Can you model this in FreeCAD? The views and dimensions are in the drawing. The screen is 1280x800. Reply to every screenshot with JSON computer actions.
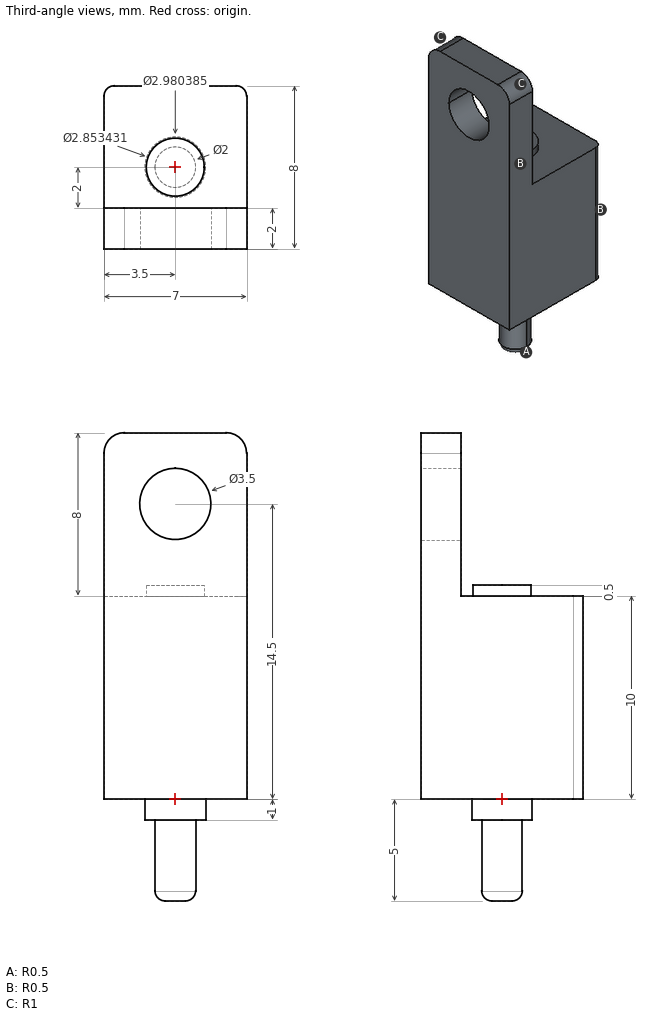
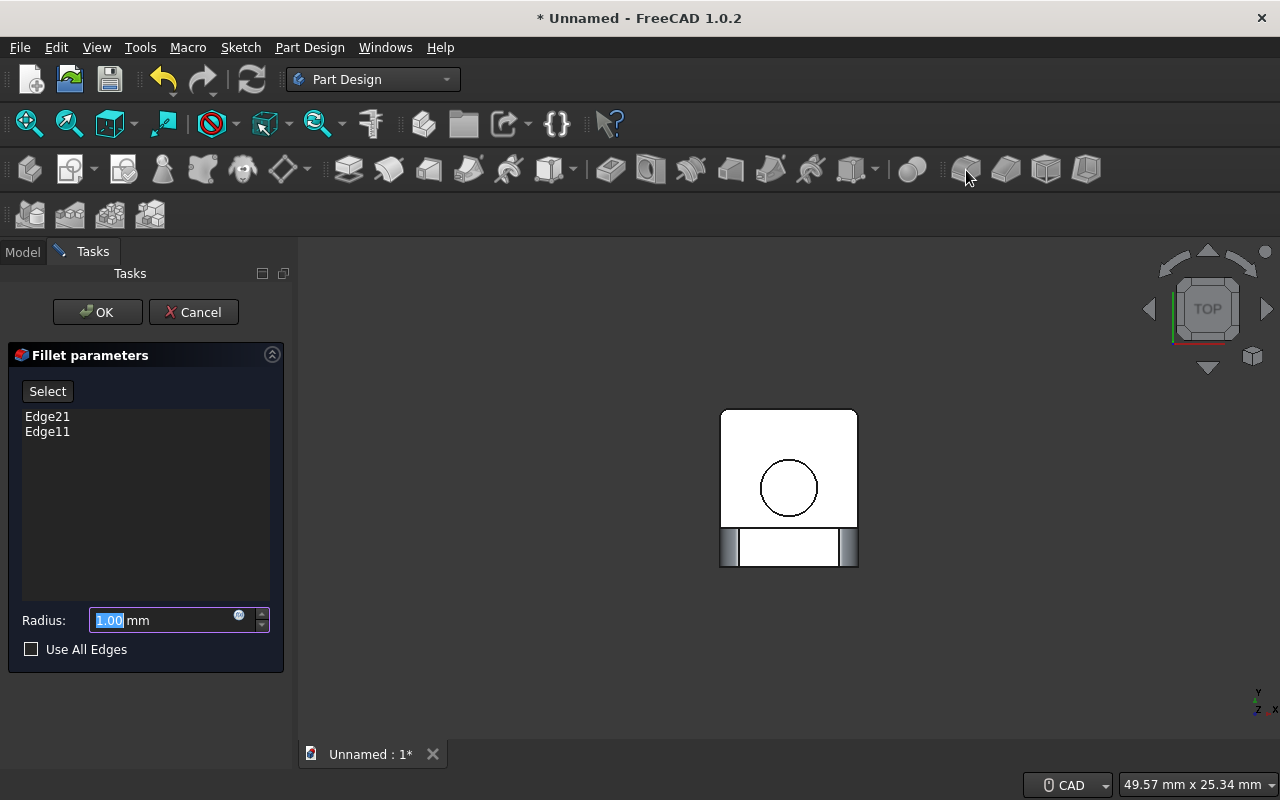
{"action": "type", "text": "1"}
{"action": "key", "text": "Tab"}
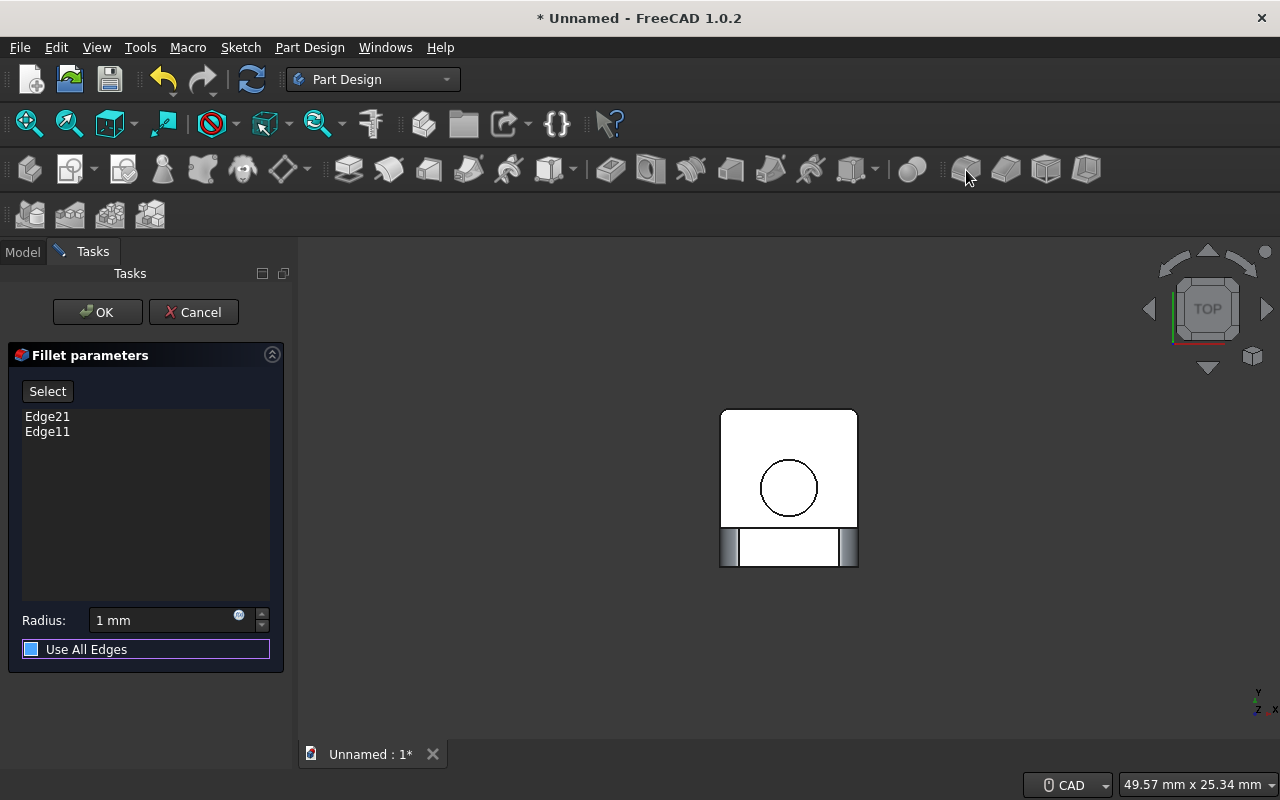
{"action": "left_click", "coordinate": [98, 312]}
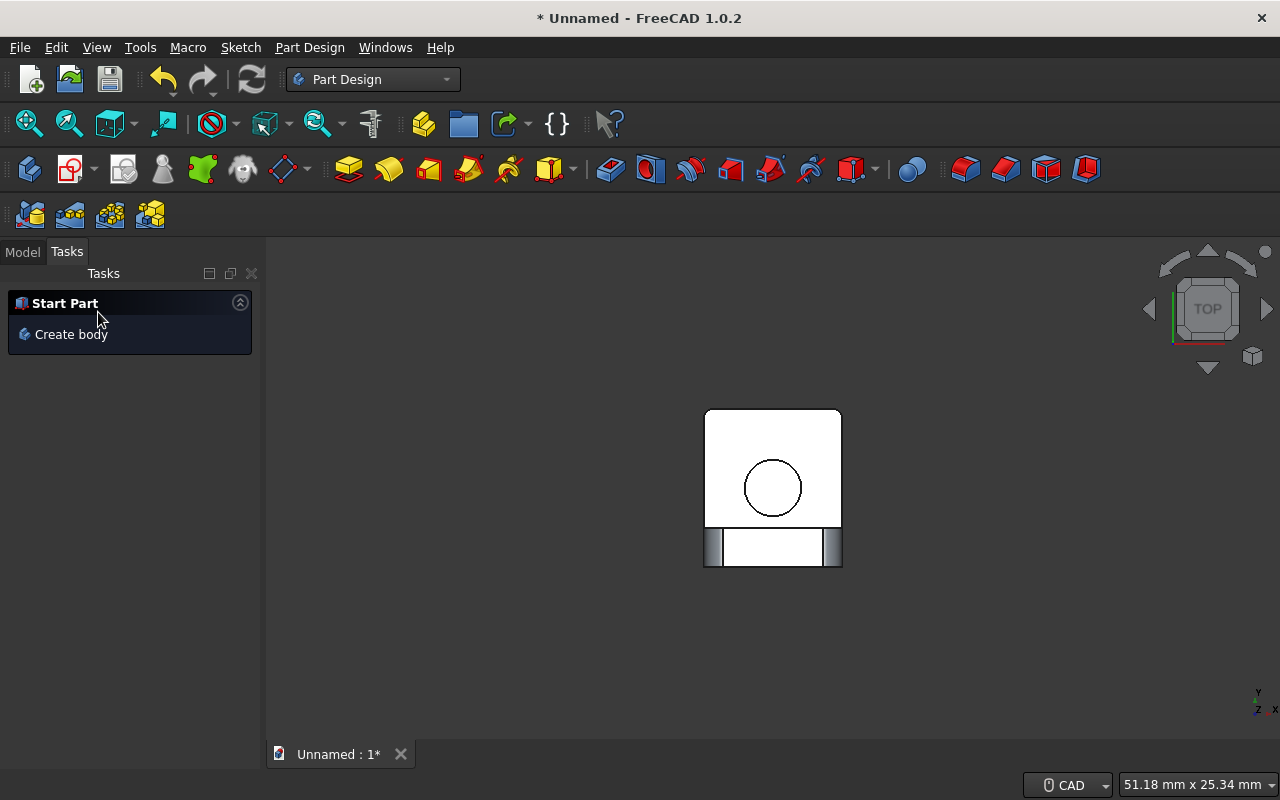
{"action": "left_click", "coordinate": [30, 124]}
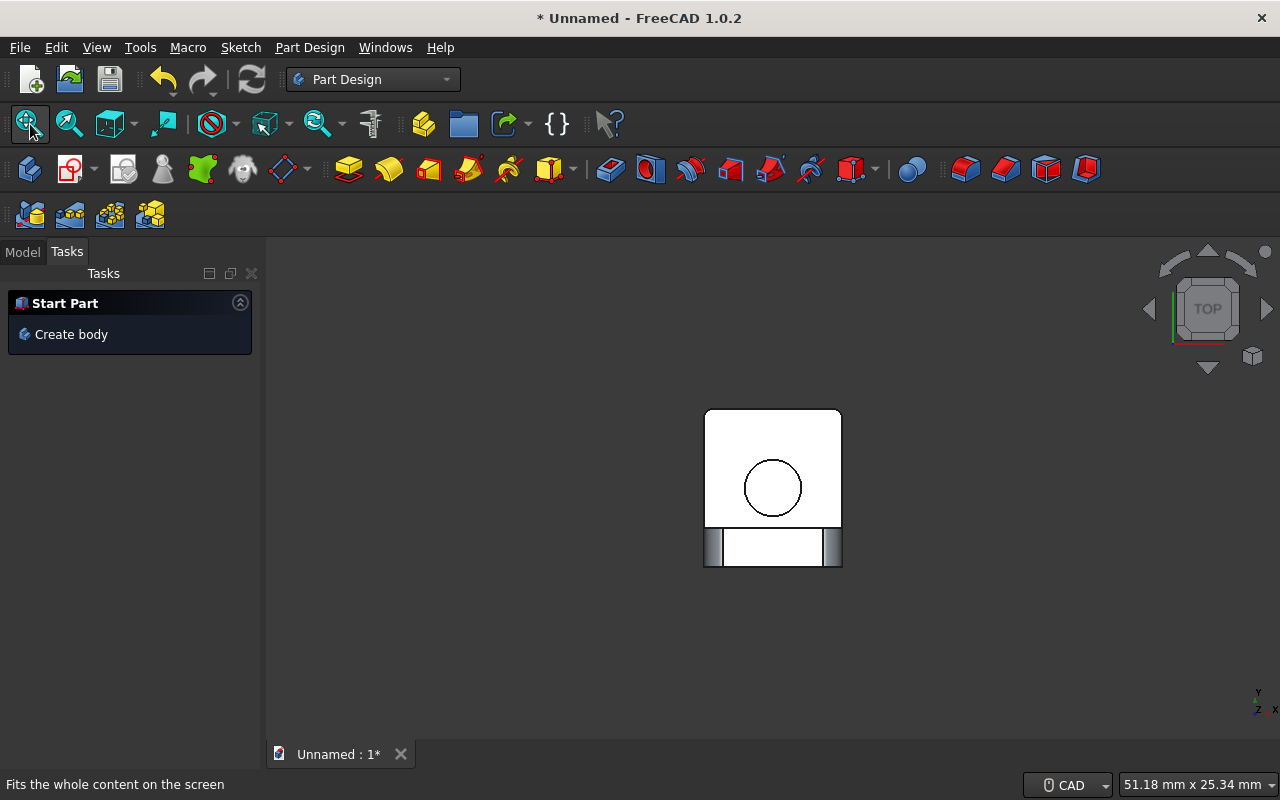
{"action": "key", "text": "4"}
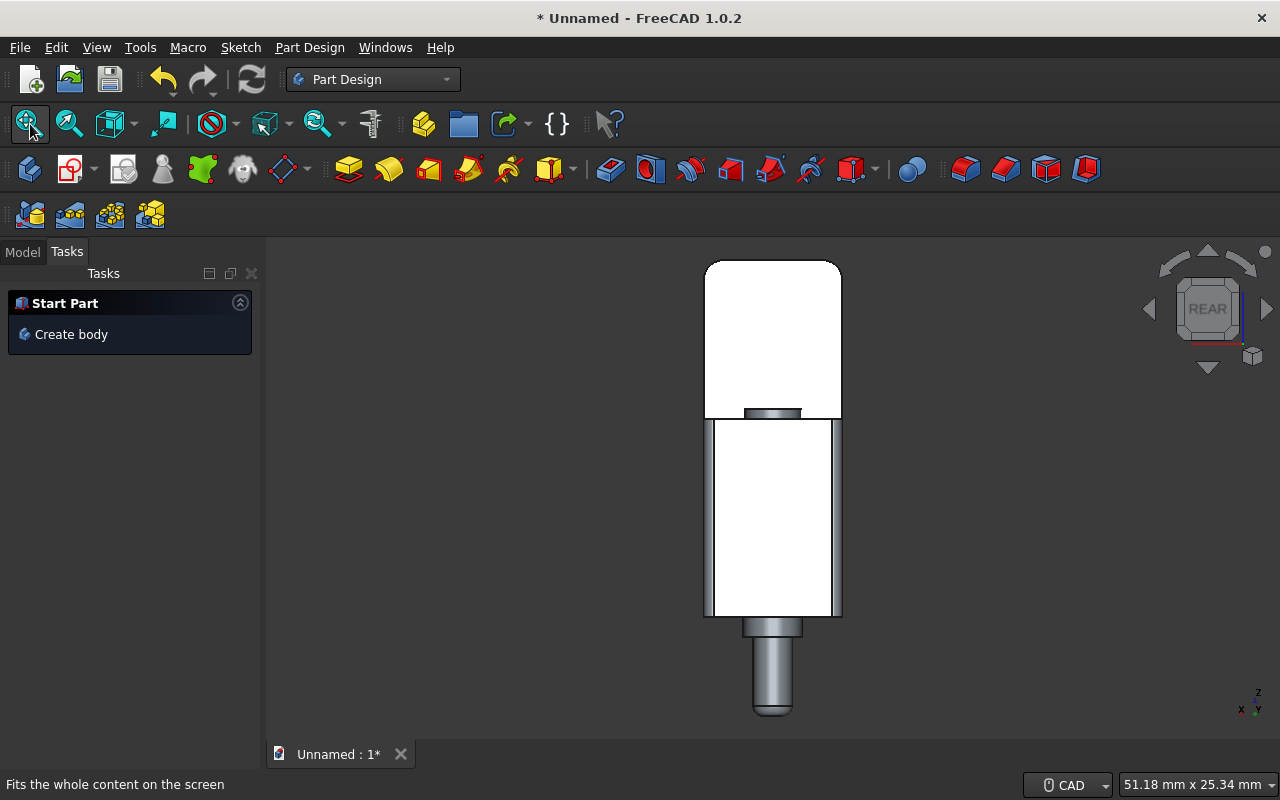
{"action": "left_click", "coordinate": [773, 338]}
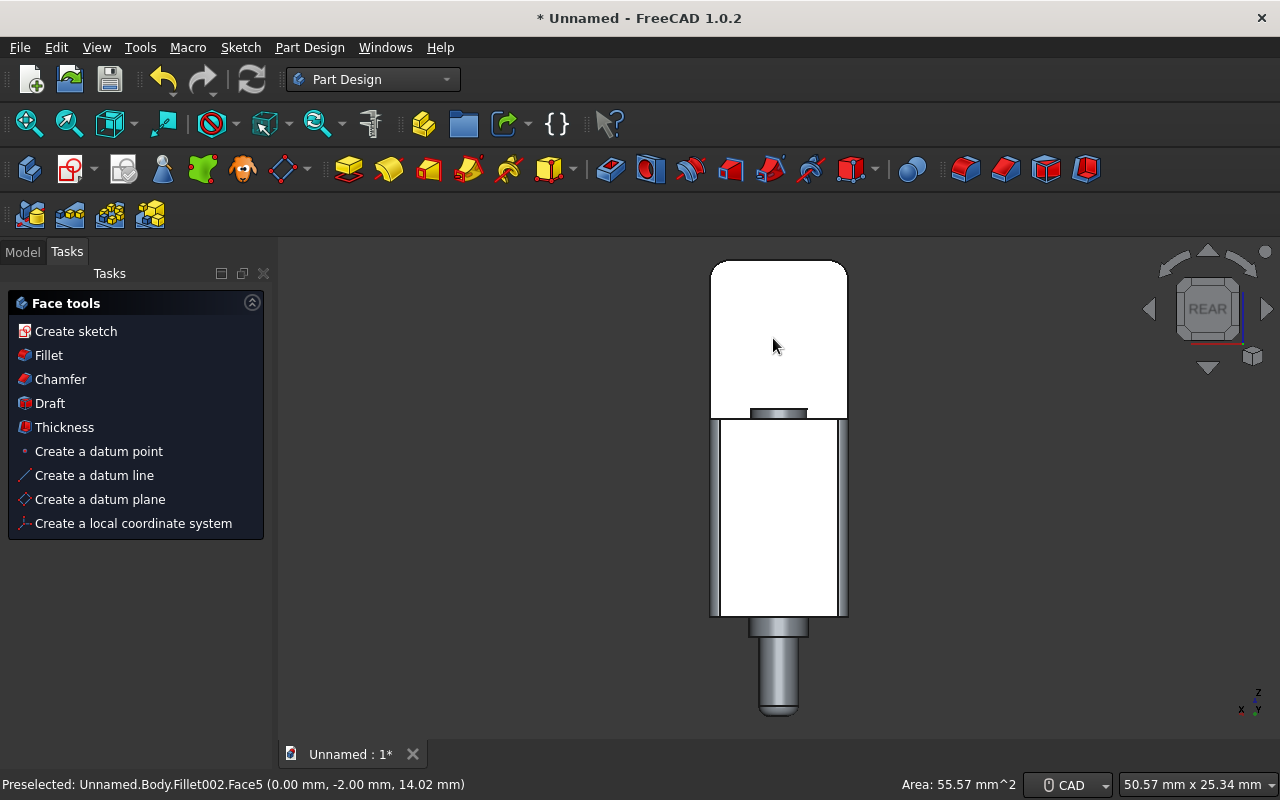
{"action": "left_click", "coordinate": [70, 170]}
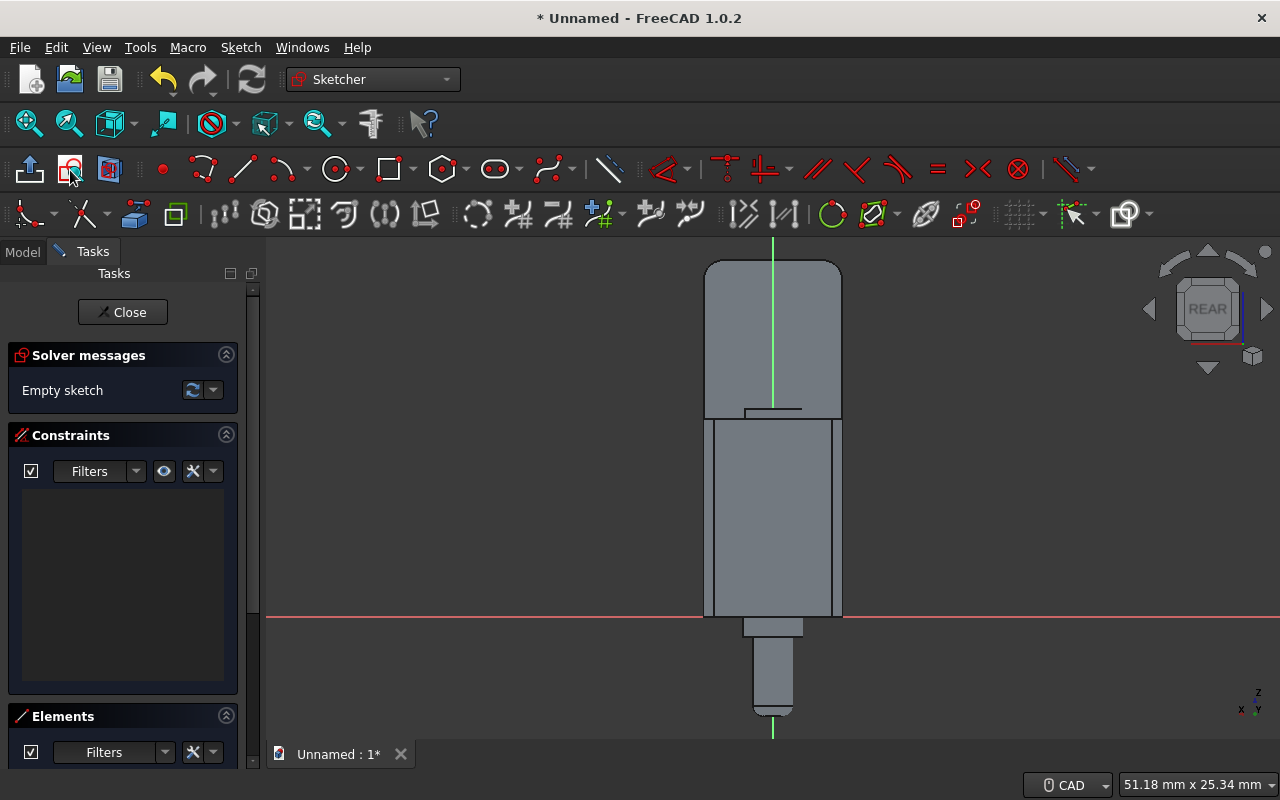
{"action": "scroll", "coordinate": [790, 289], "scroll_direction": "up", "scroll_amount": 8}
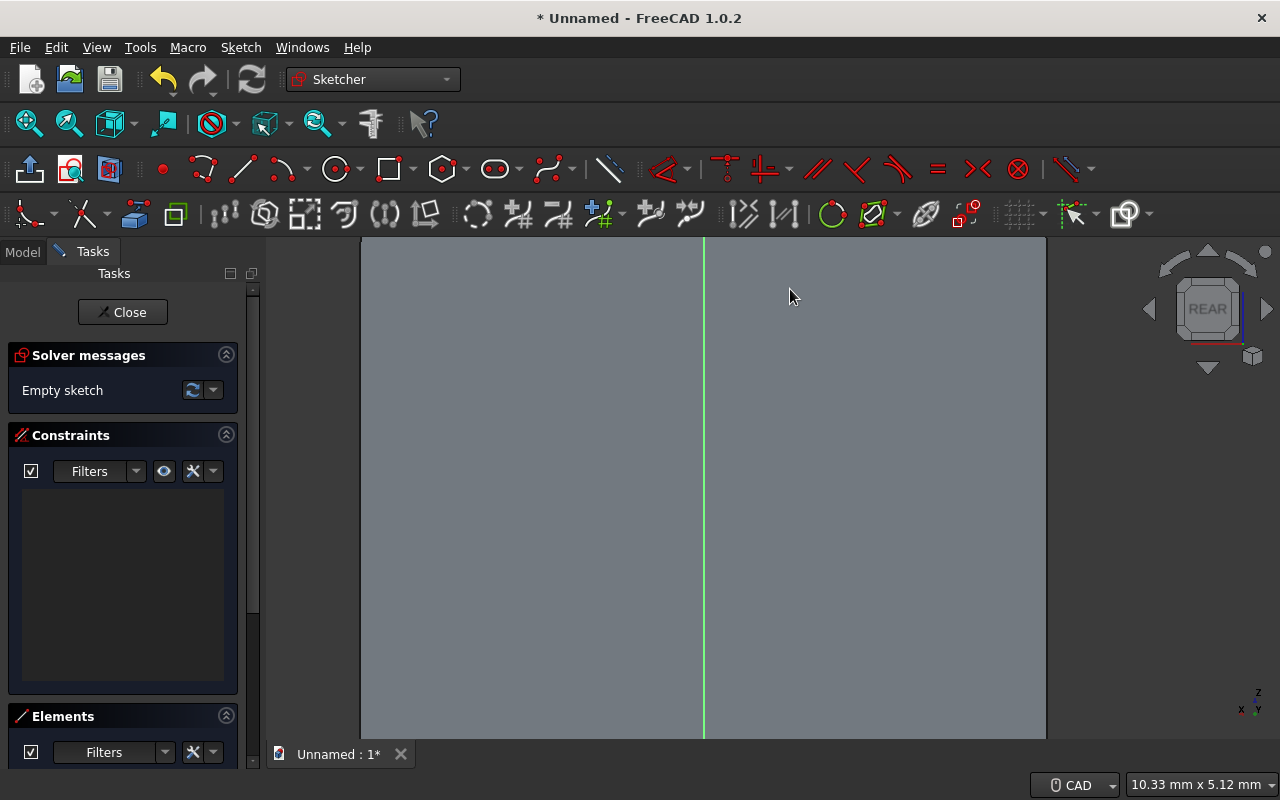
{"action": "key", "text": "g c"}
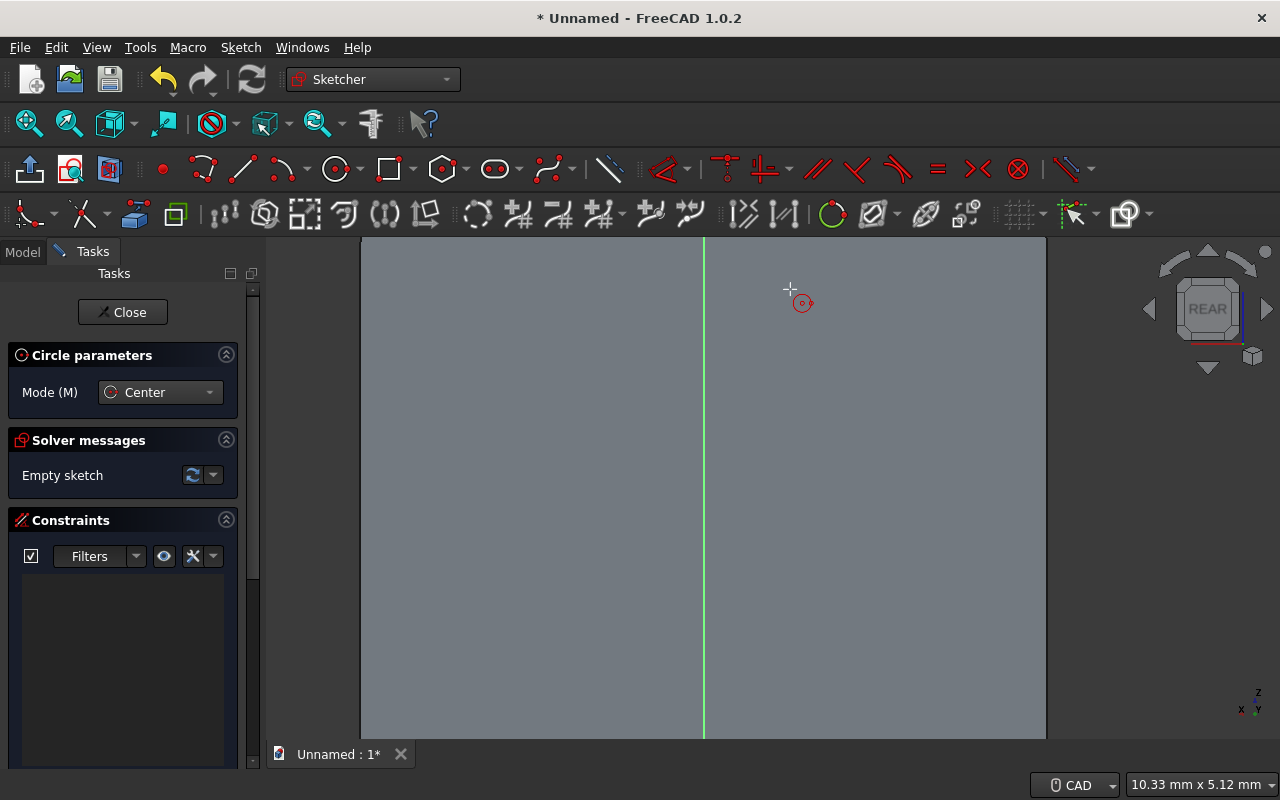
{"action": "left_click", "coordinate": [704, 489]}
{"action": "mouse_move", "coordinate": [825, 368]}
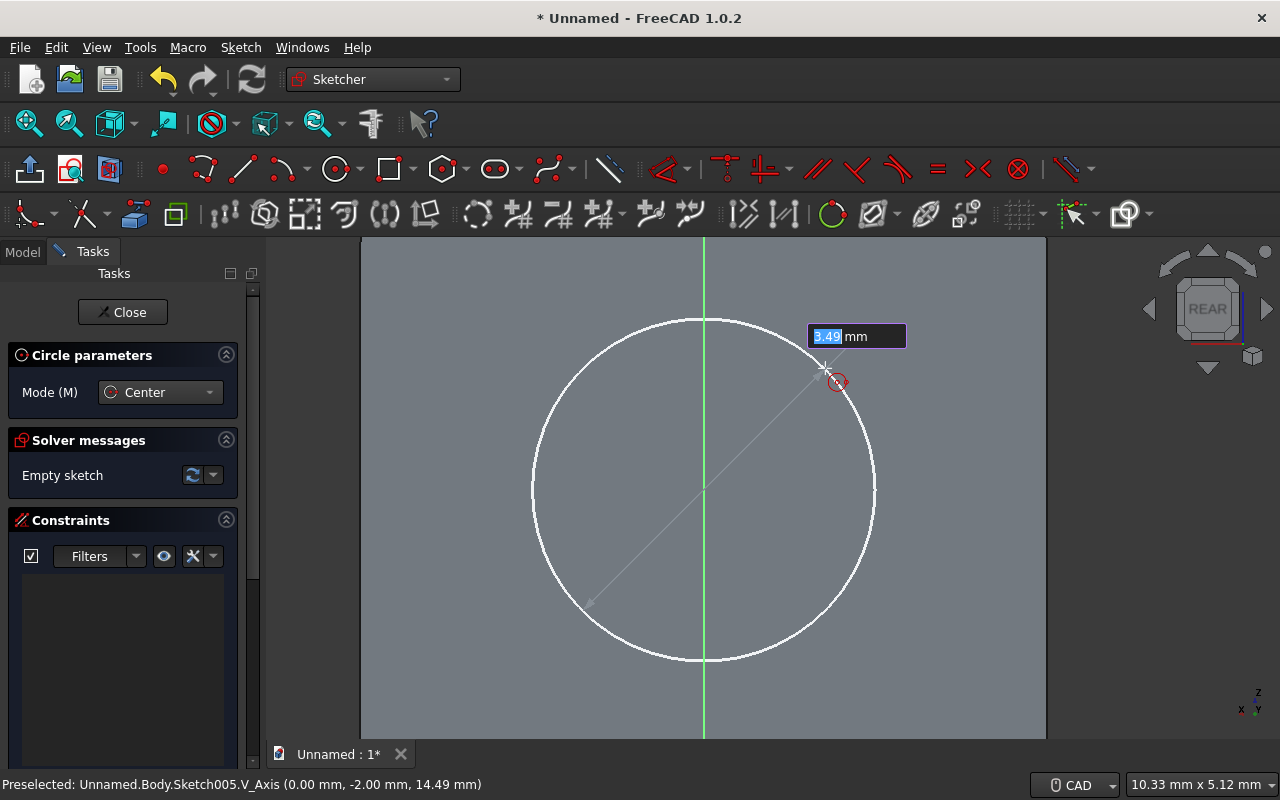
{"action": "type", "text": "3.5"}
{"action": "key", "text": "Return"}
{"action": "key", "text": "Escape"}